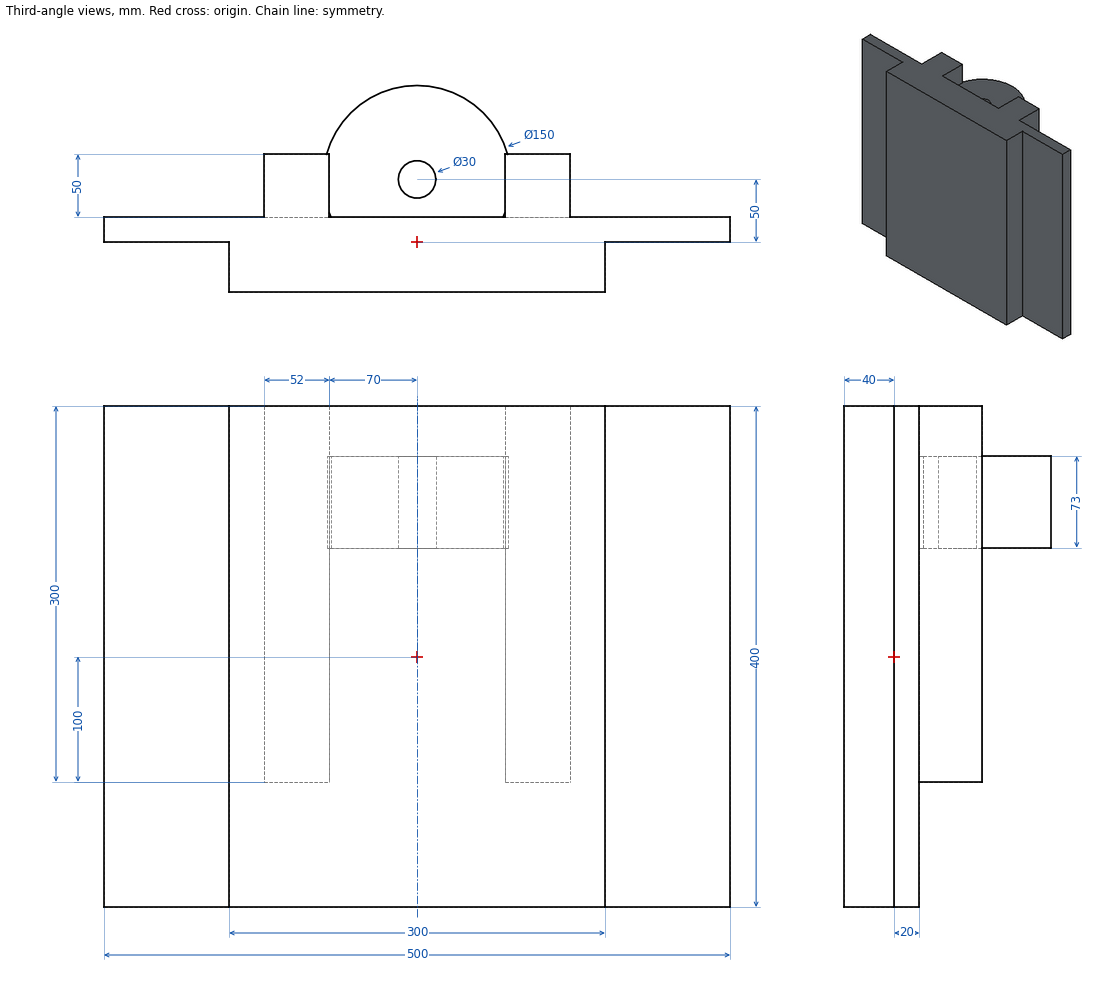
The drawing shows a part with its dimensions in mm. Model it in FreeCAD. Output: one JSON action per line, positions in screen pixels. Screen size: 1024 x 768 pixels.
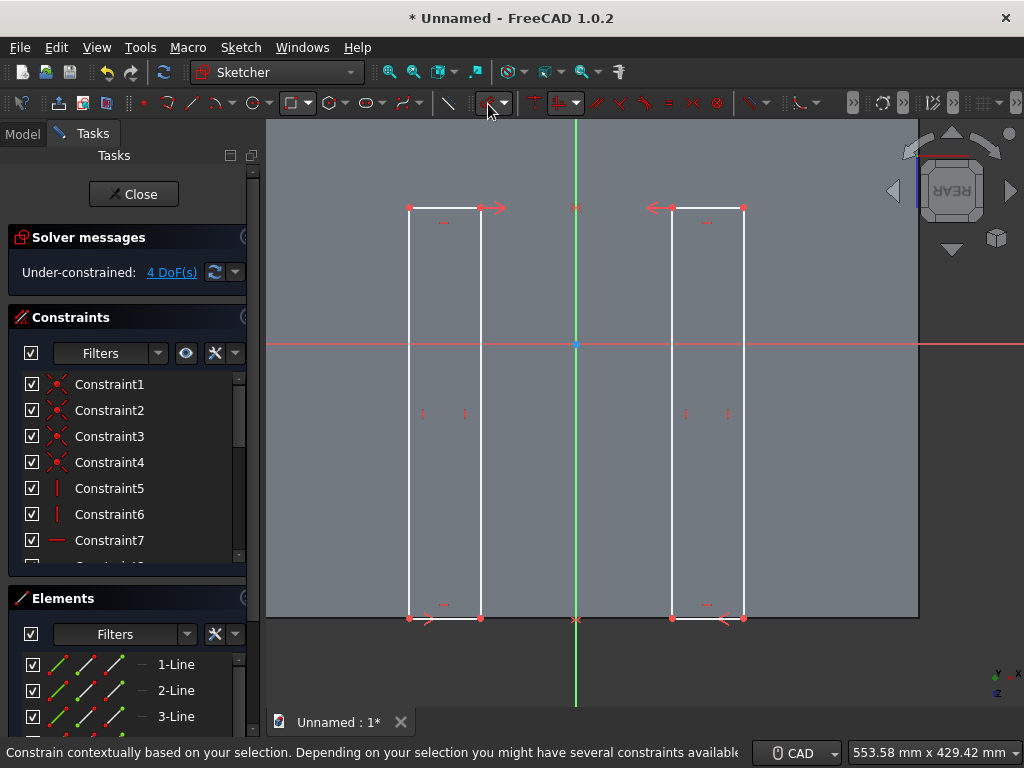
{"action": "left_click", "coordinate": [431, 619]}
{"action": "left_click", "coordinate": [445, 653]}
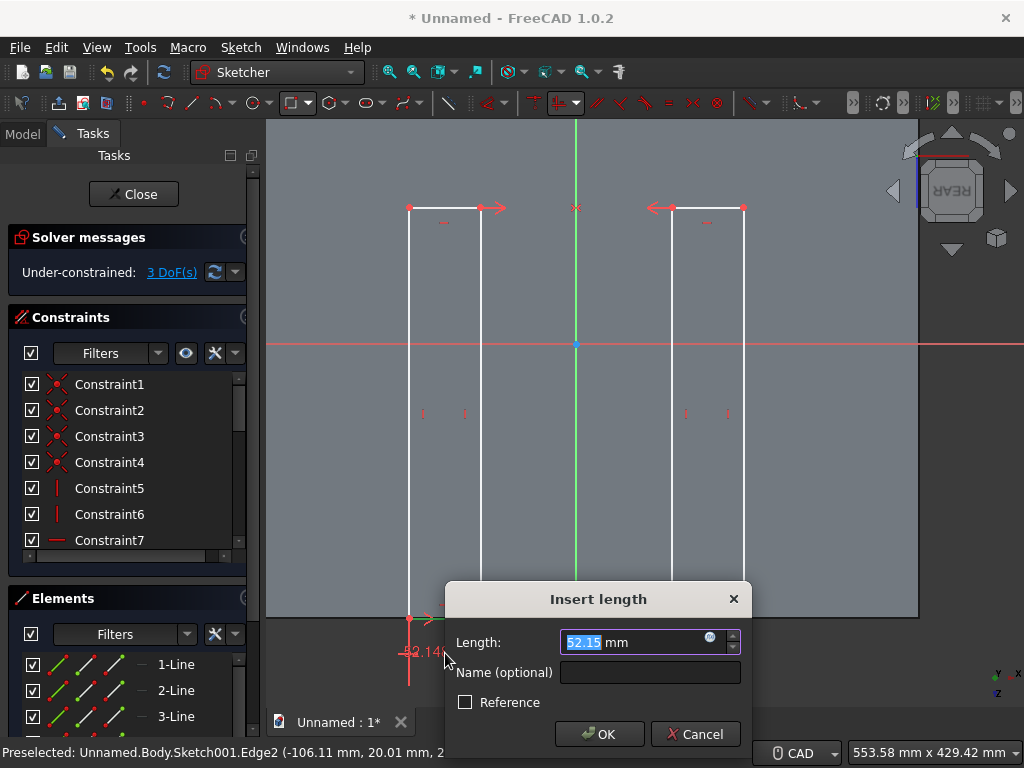
{"action": "type", "text": "52"}
{"action": "key", "text": "Return"}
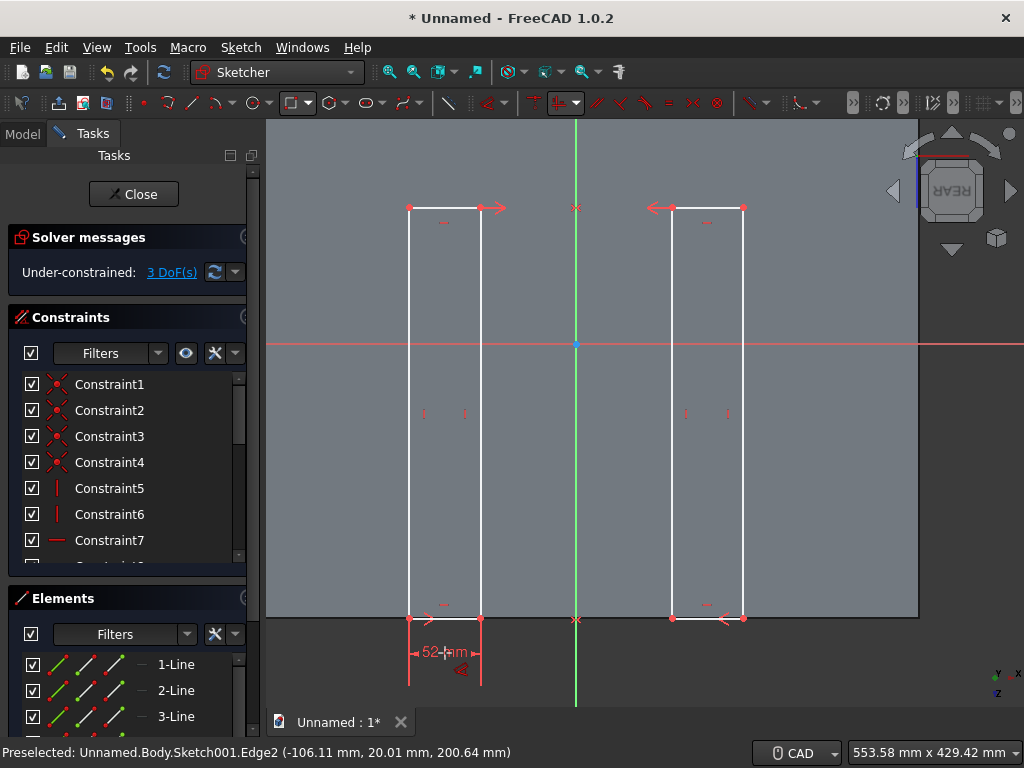
{"action": "left_click", "coordinate": [409, 331]}
{"action": "left_click", "coordinate": [375, 414]}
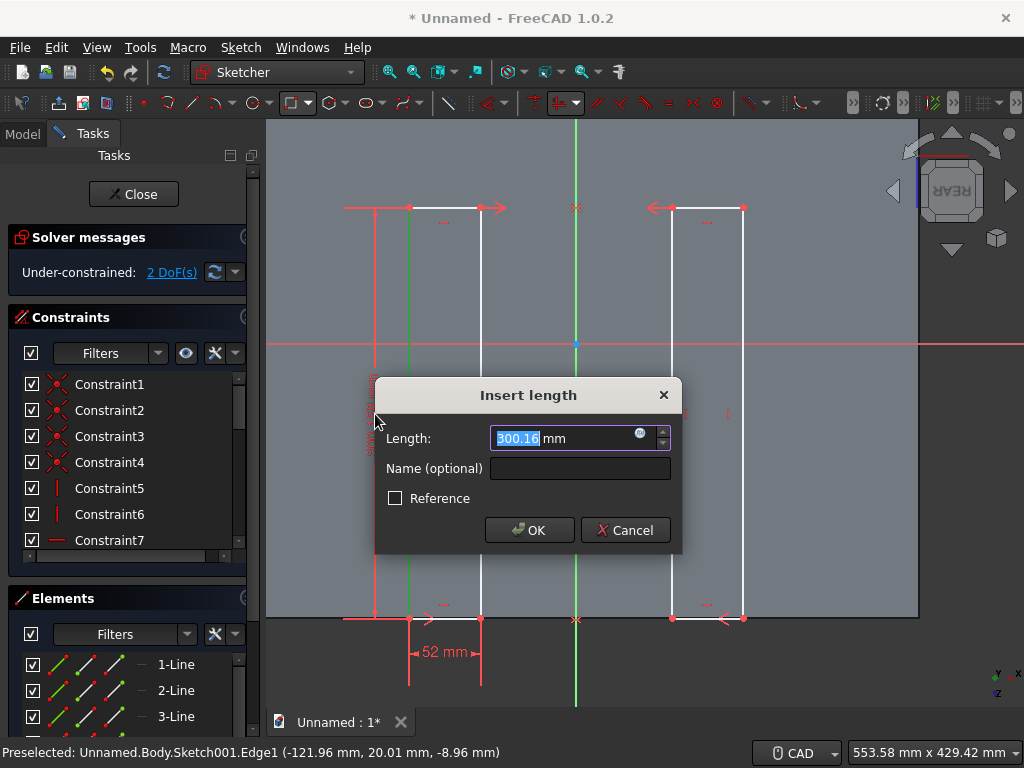
{"action": "type", "text": "300"}
{"action": "key", "text": "Return"}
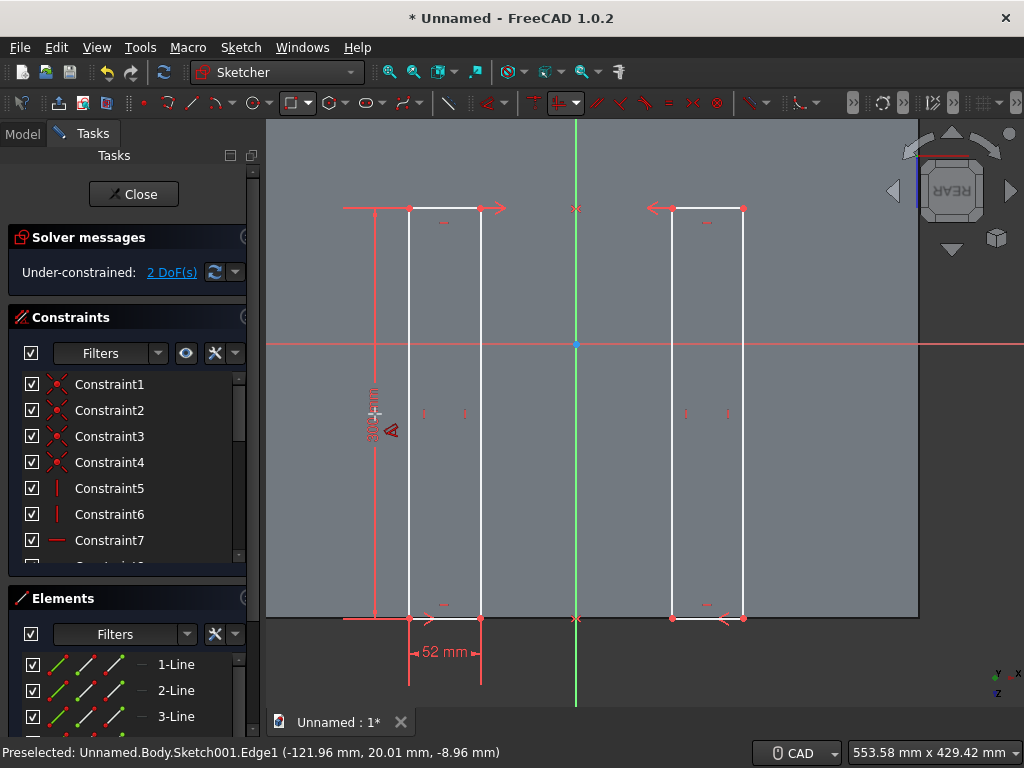
{"action": "left_click", "coordinate": [481, 619]}
{"action": "left_click", "coordinate": [528, 653]}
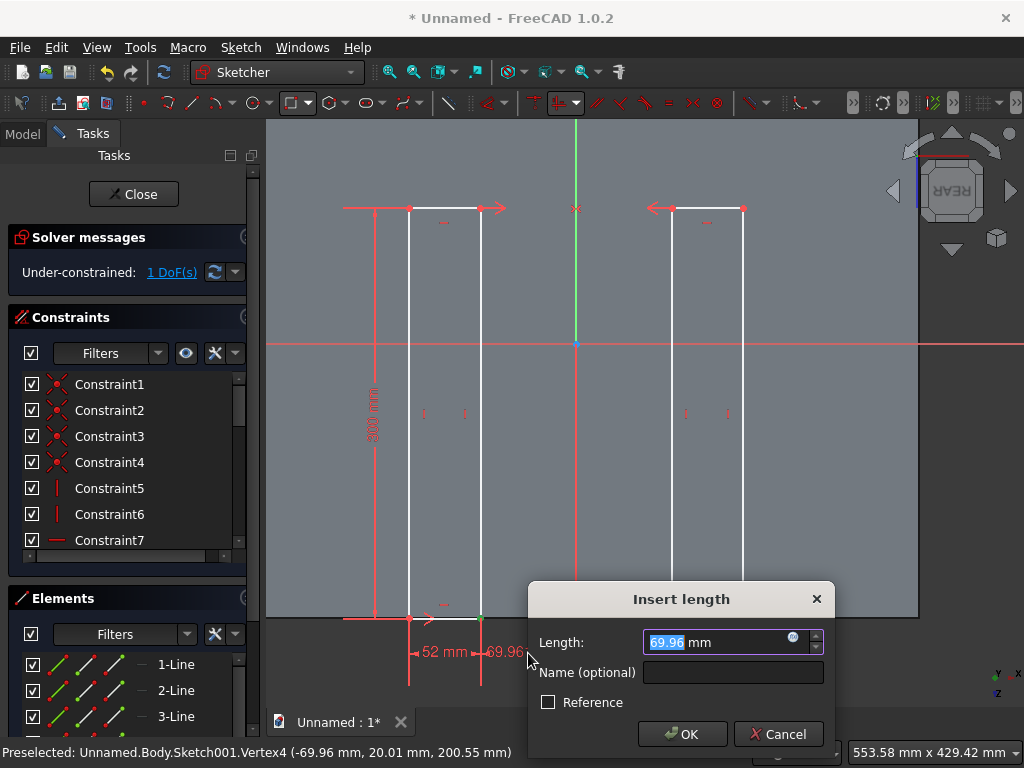
{"action": "type", "text": "70"}
{"action": "key", "text": "Return"}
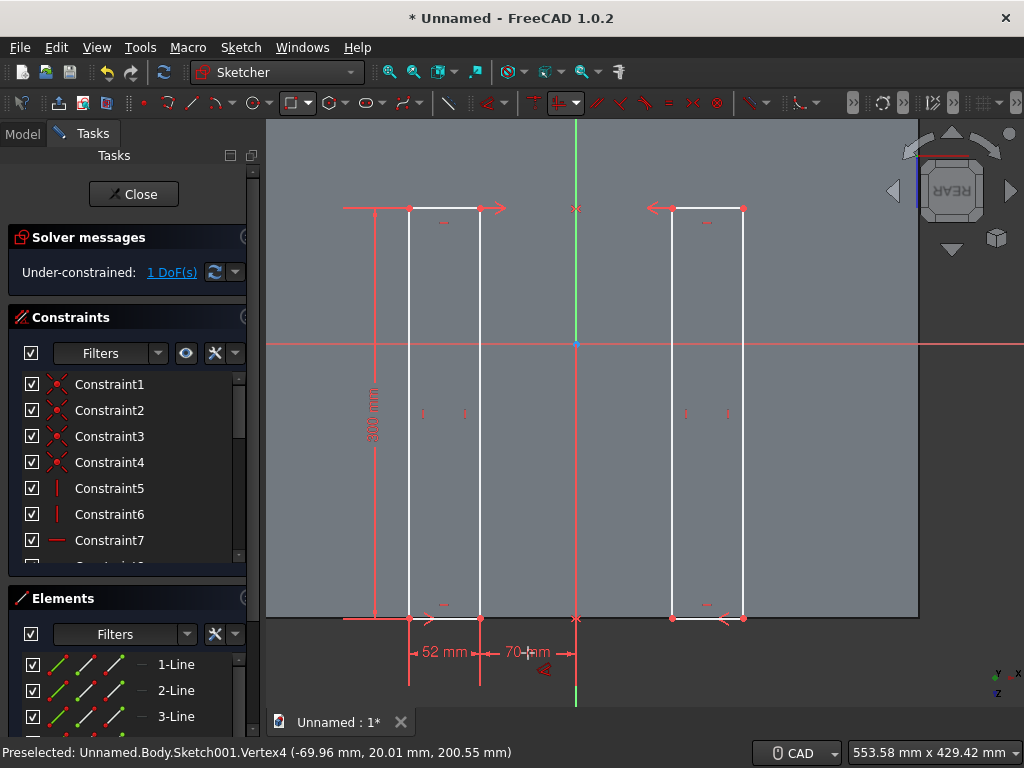
{"action": "left_click", "coordinate": [409, 208]}
{"action": "left_click", "coordinate": [375, 276]}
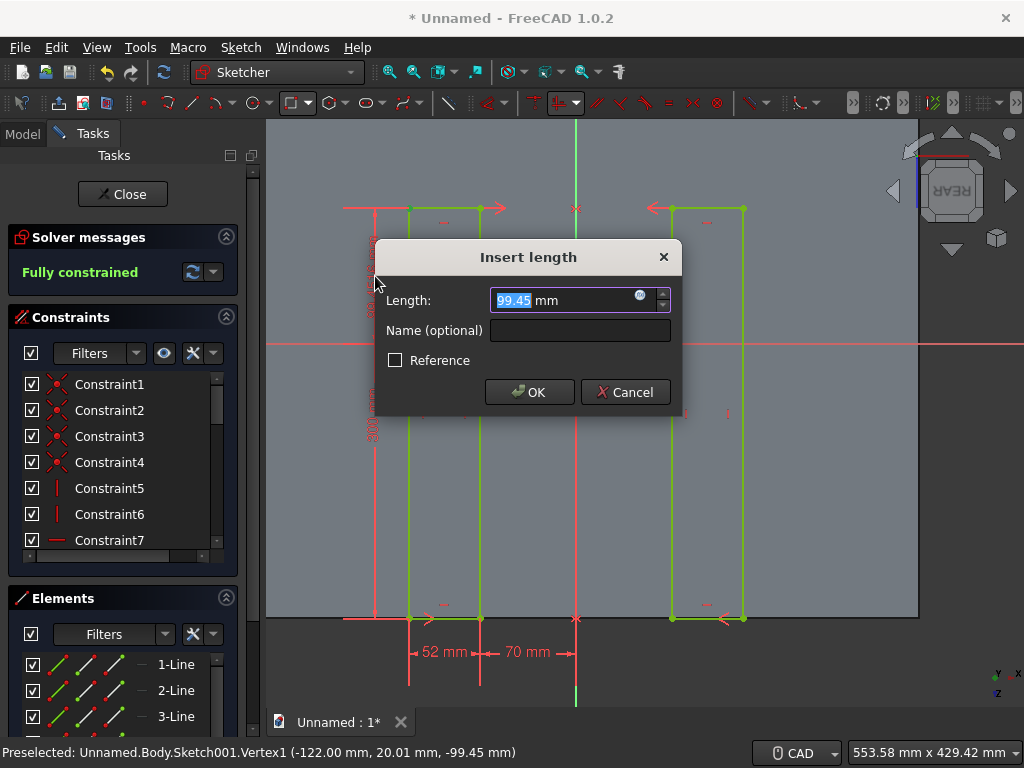
{"action": "type", "text": "100"}
{"action": "key", "text": "Return"}
{"action": "key", "text": "Escape"}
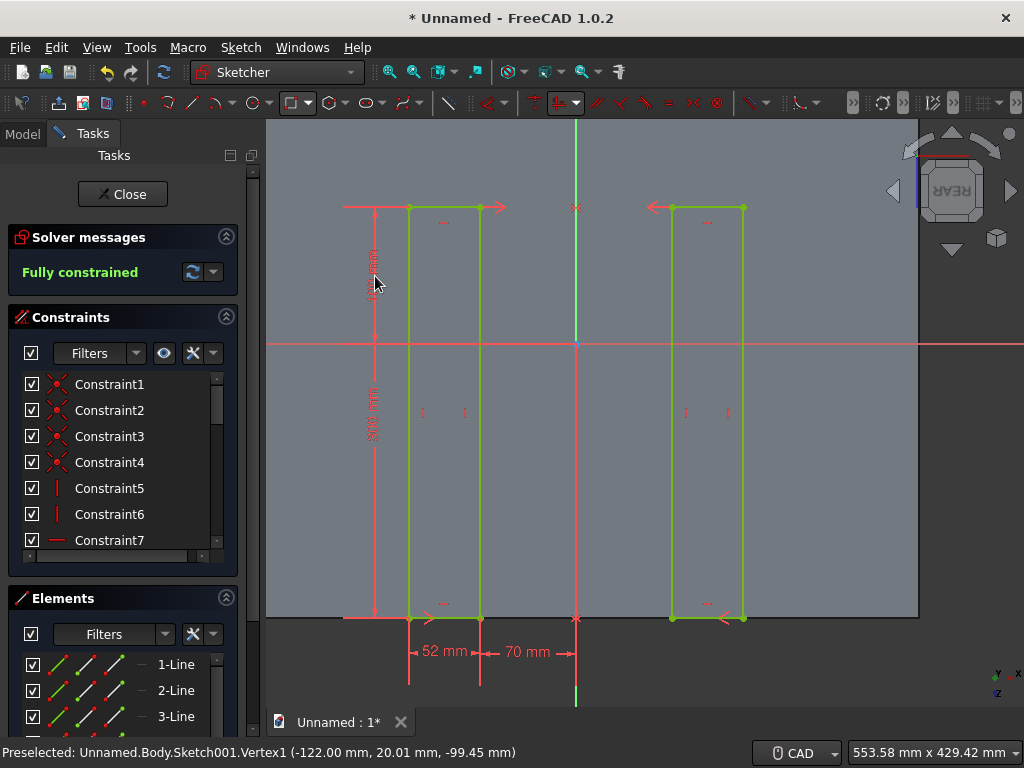
{"action": "left_click", "coordinate": [123, 194]}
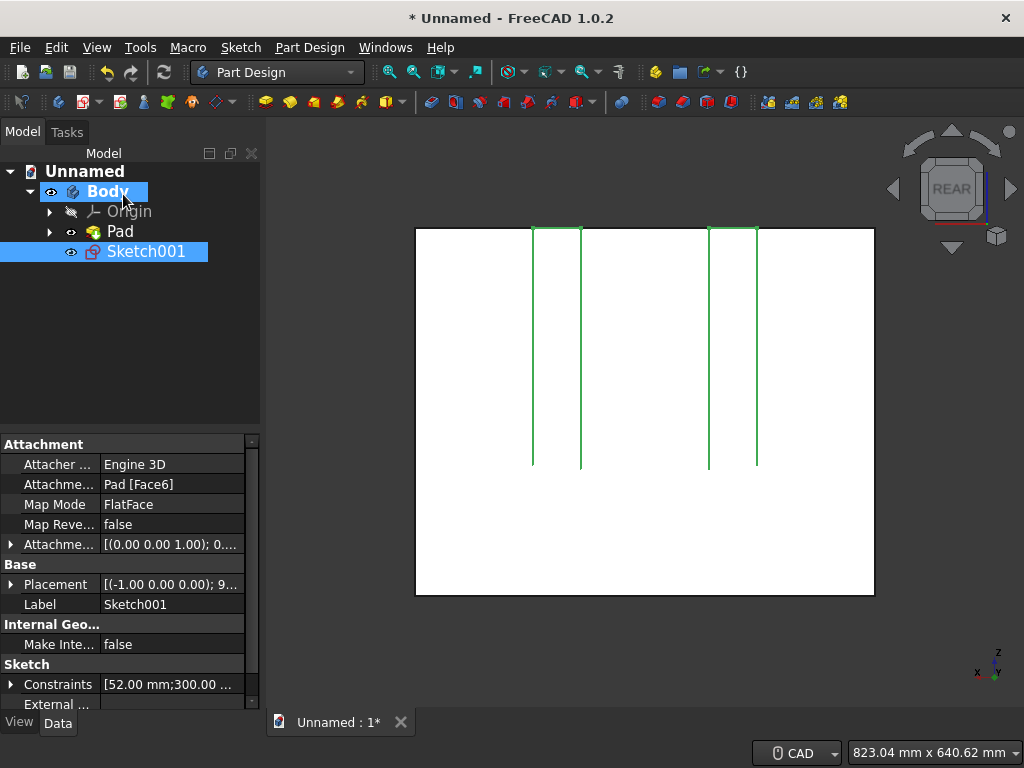
{"action": "left_click", "coordinate": [266, 102]}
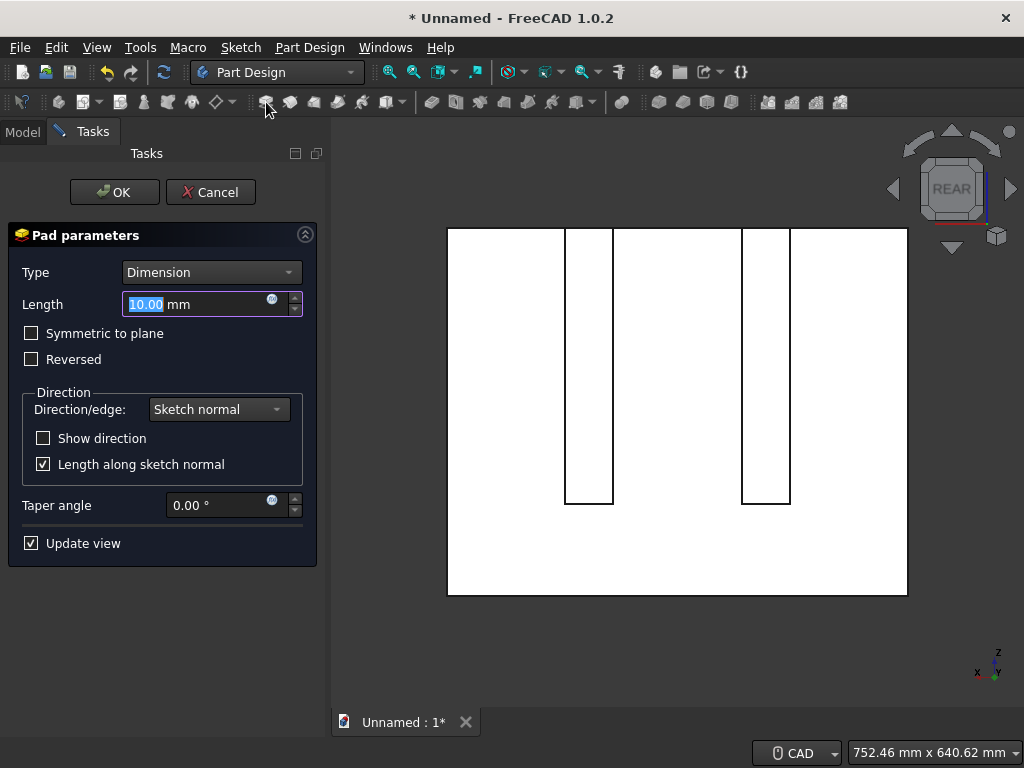
{"action": "type", "text": "50"}
{"action": "key", "text": "Tab"}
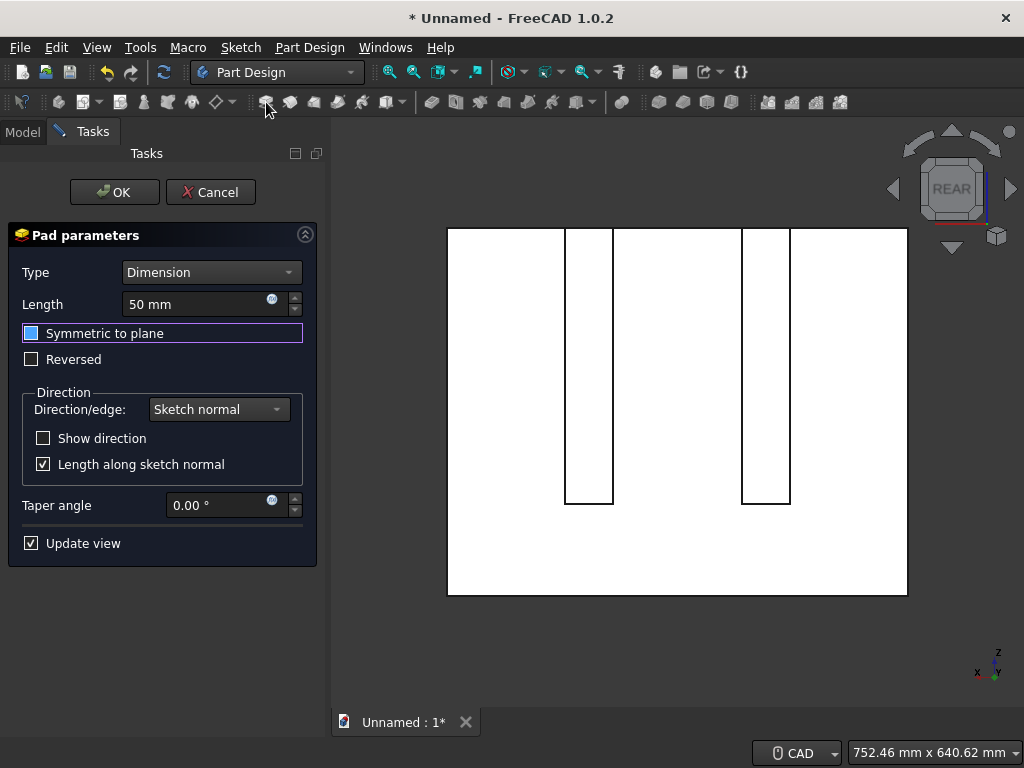
{"action": "left_click", "coordinate": [115, 192]}